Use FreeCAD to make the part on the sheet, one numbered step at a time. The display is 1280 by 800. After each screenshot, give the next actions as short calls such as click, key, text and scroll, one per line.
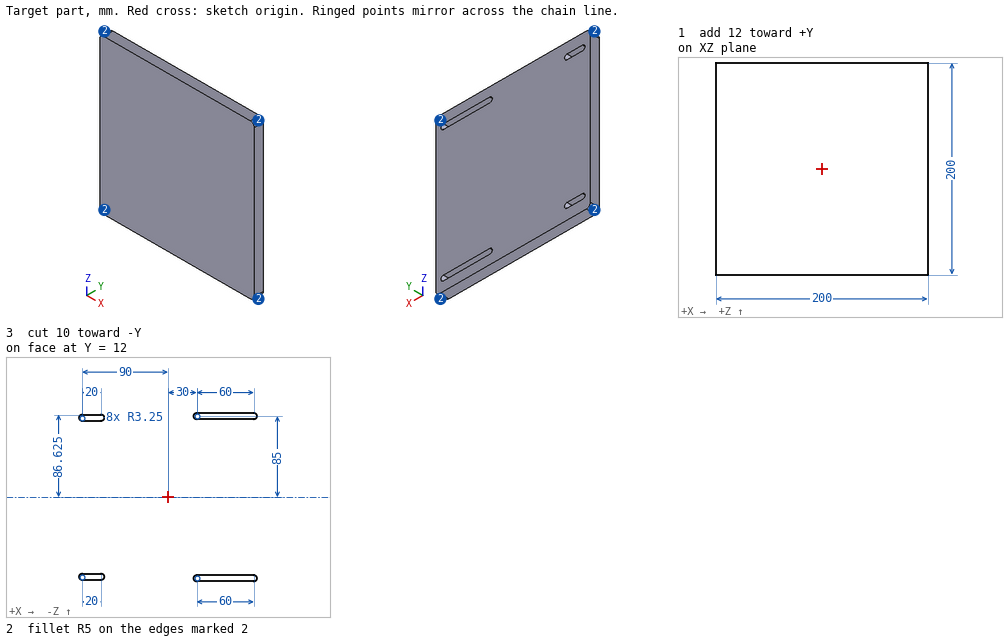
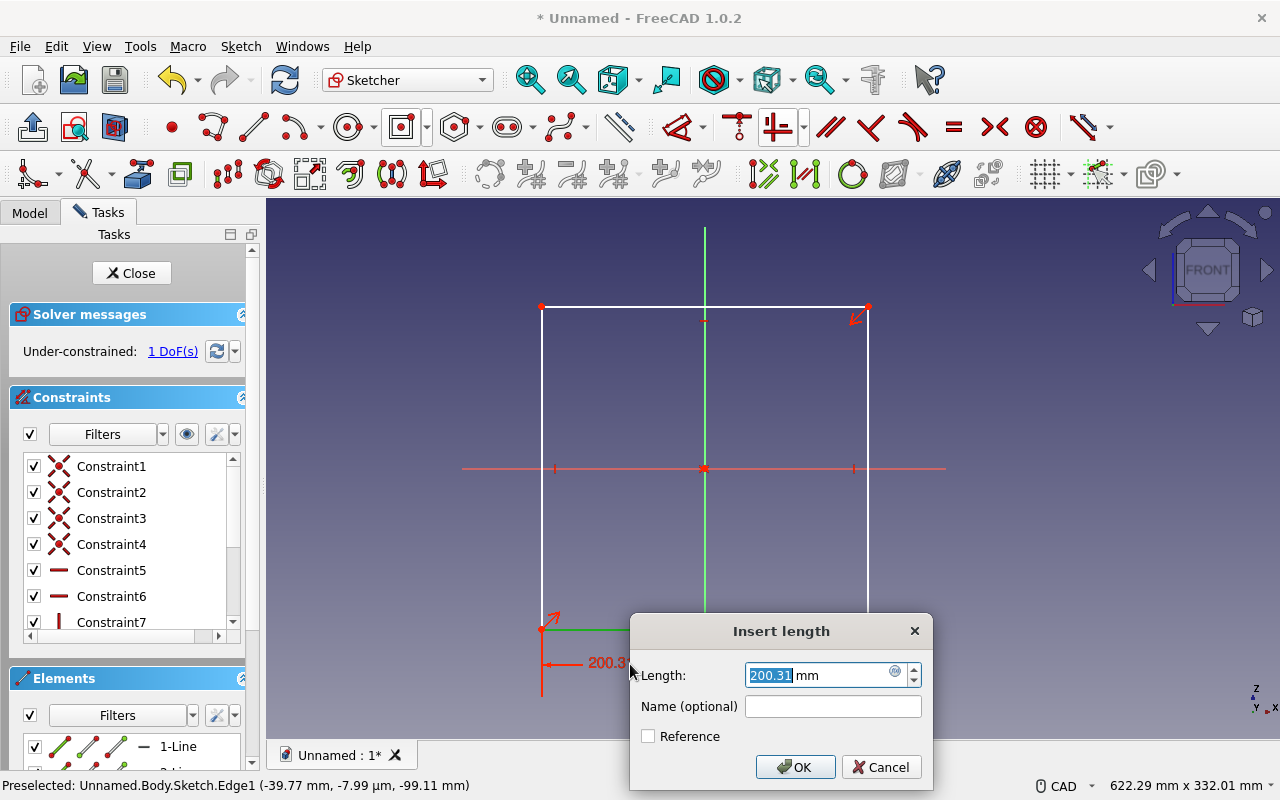
text(200)
key(Return)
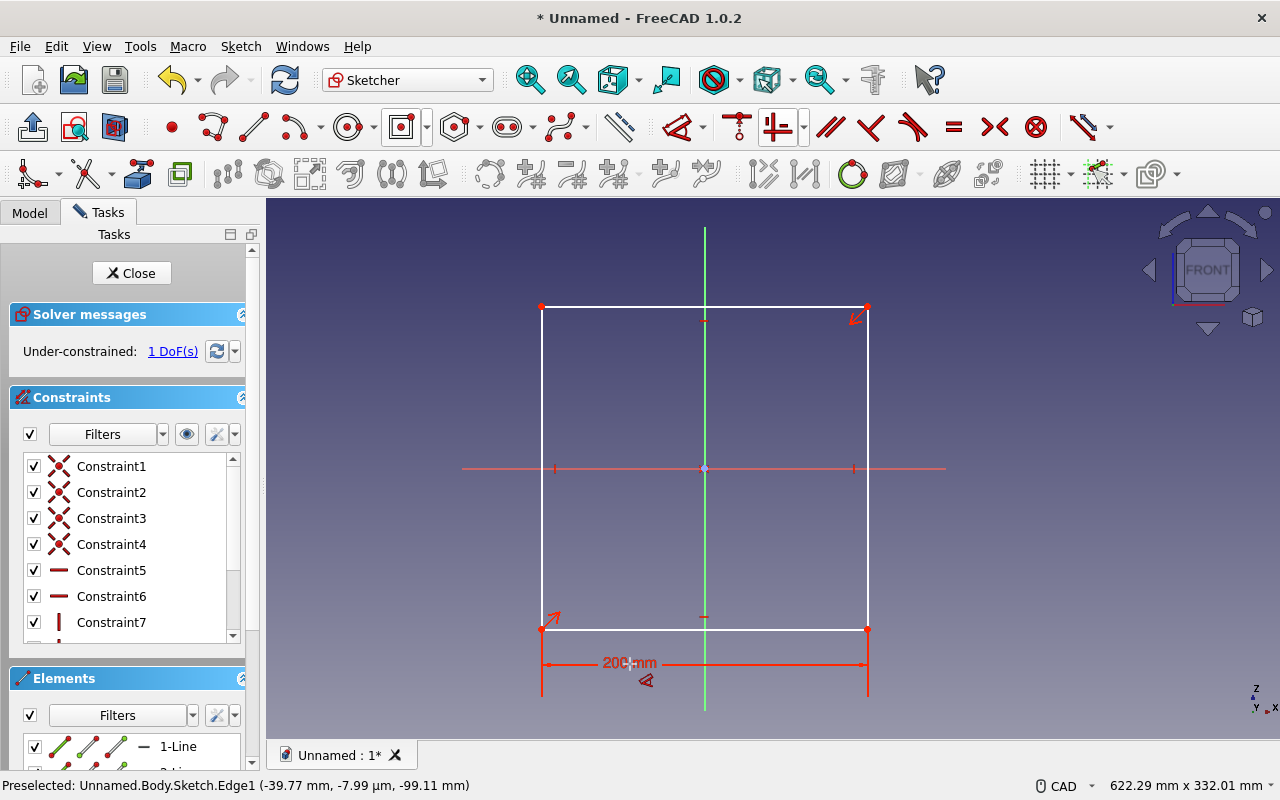
click(868, 533)
click(902, 394)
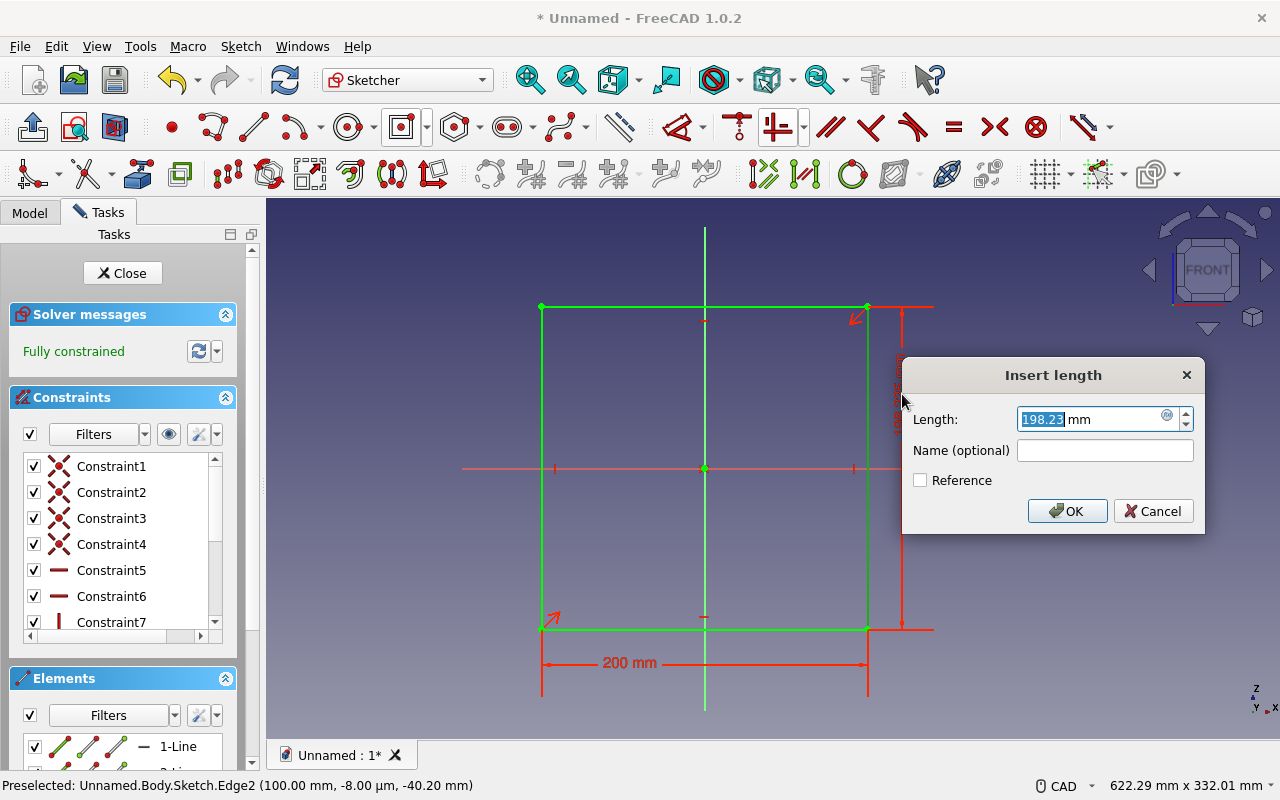
text(200)
key(Return)
key(Escape)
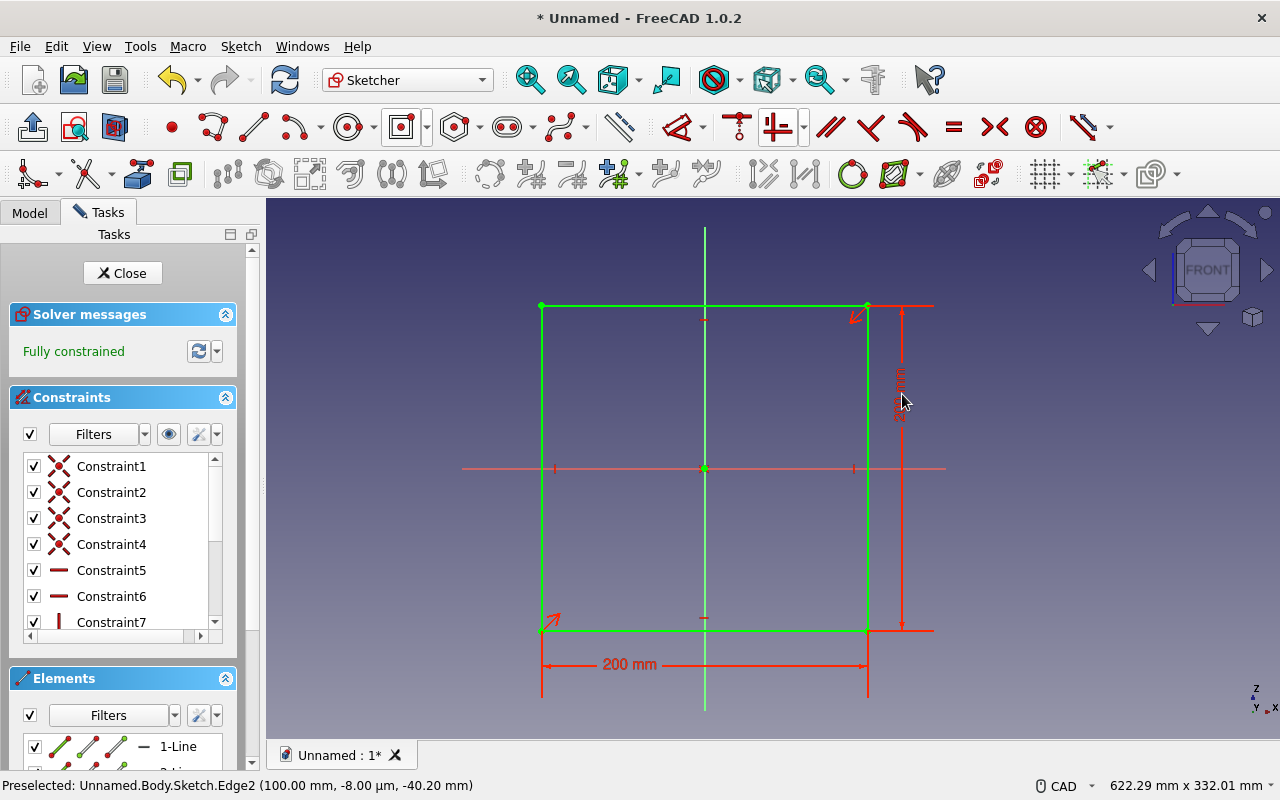
click(123, 273)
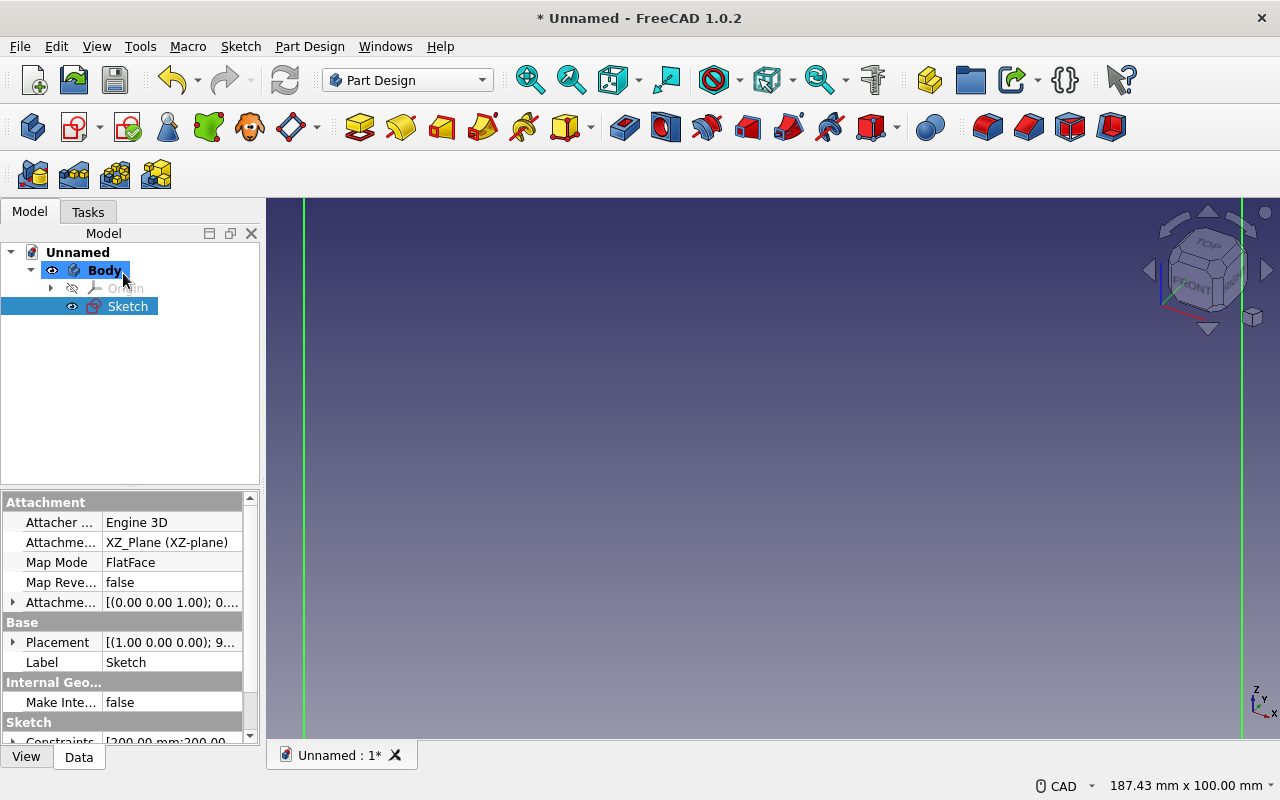
click(360, 128)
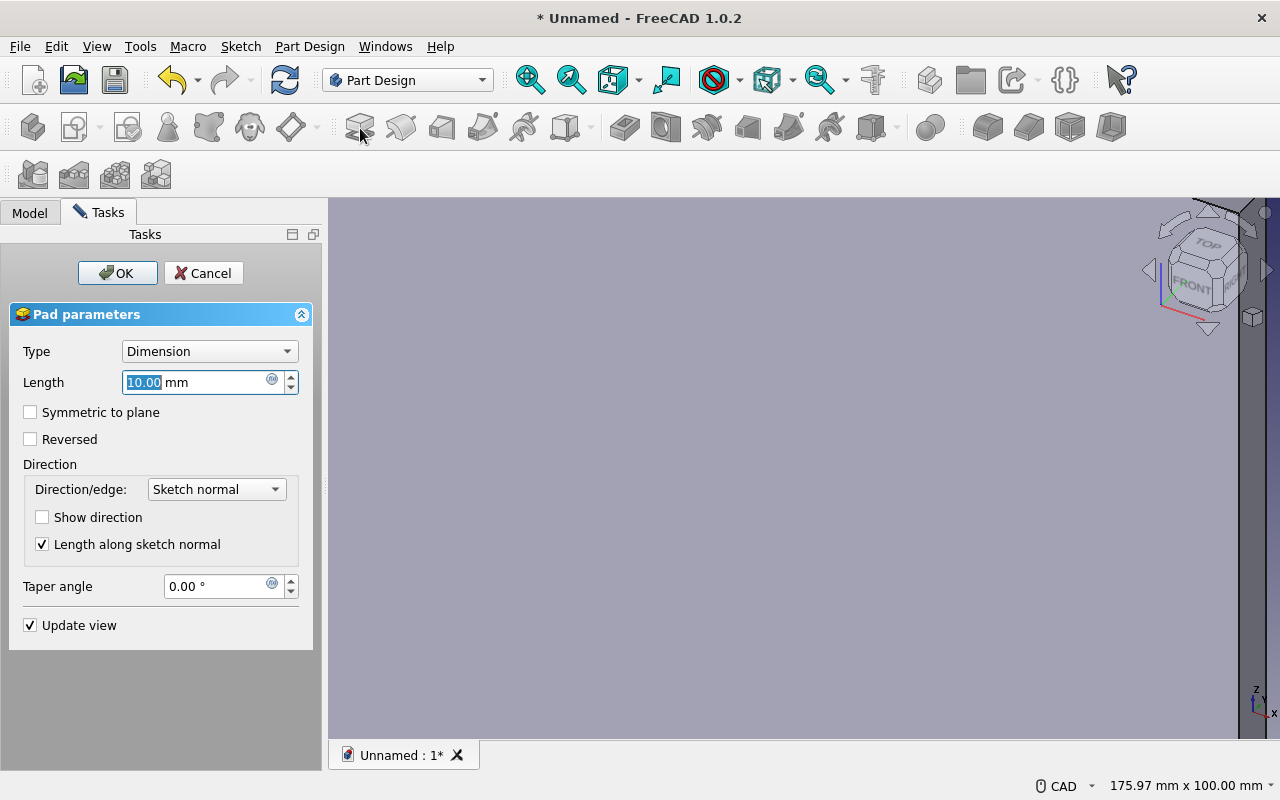
text(12)
key(Tab)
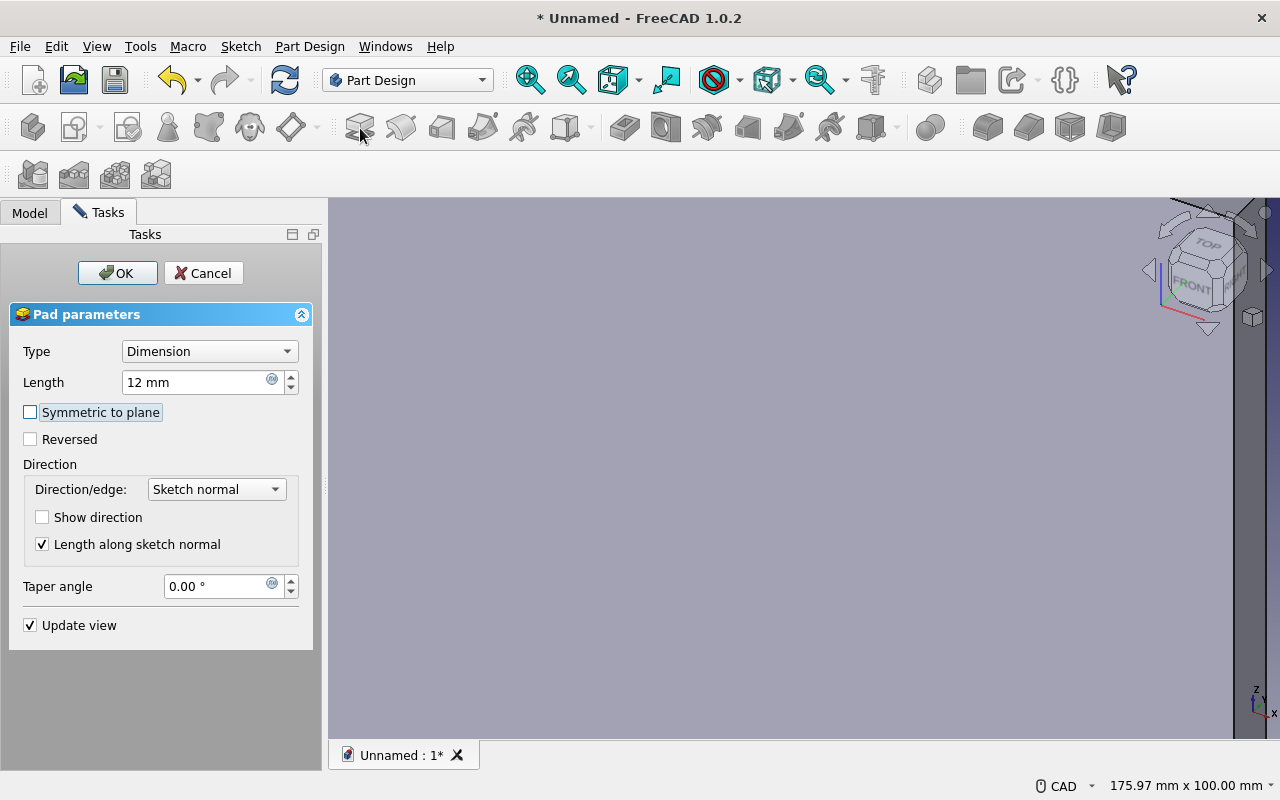
click(31, 439)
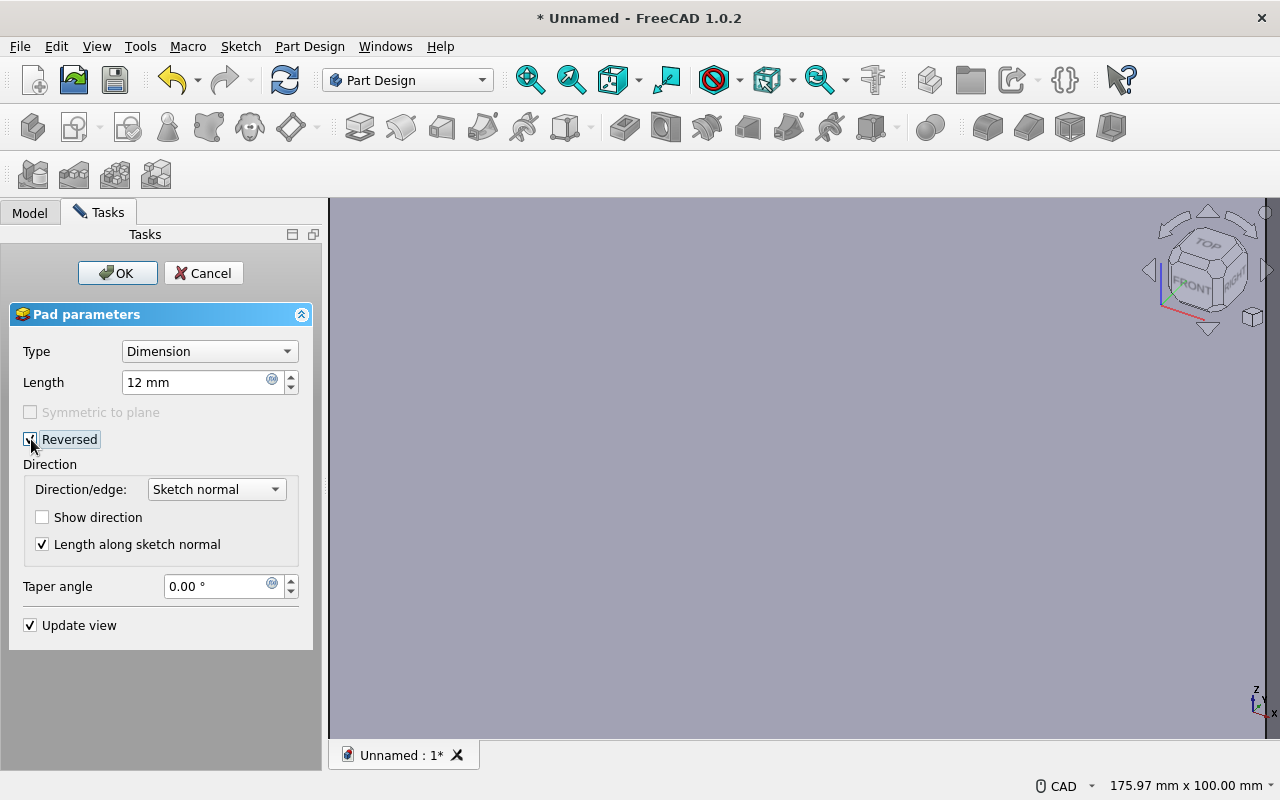
click(118, 273)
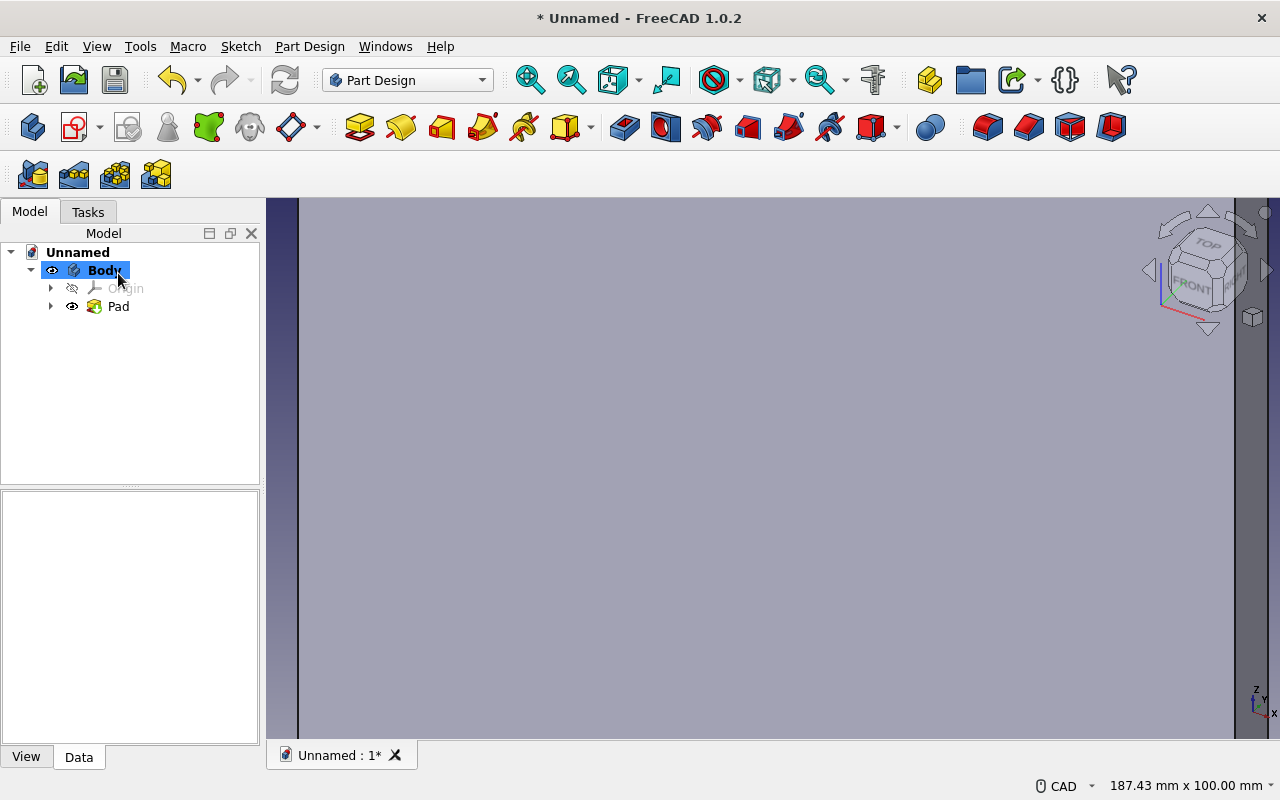
click(531, 80)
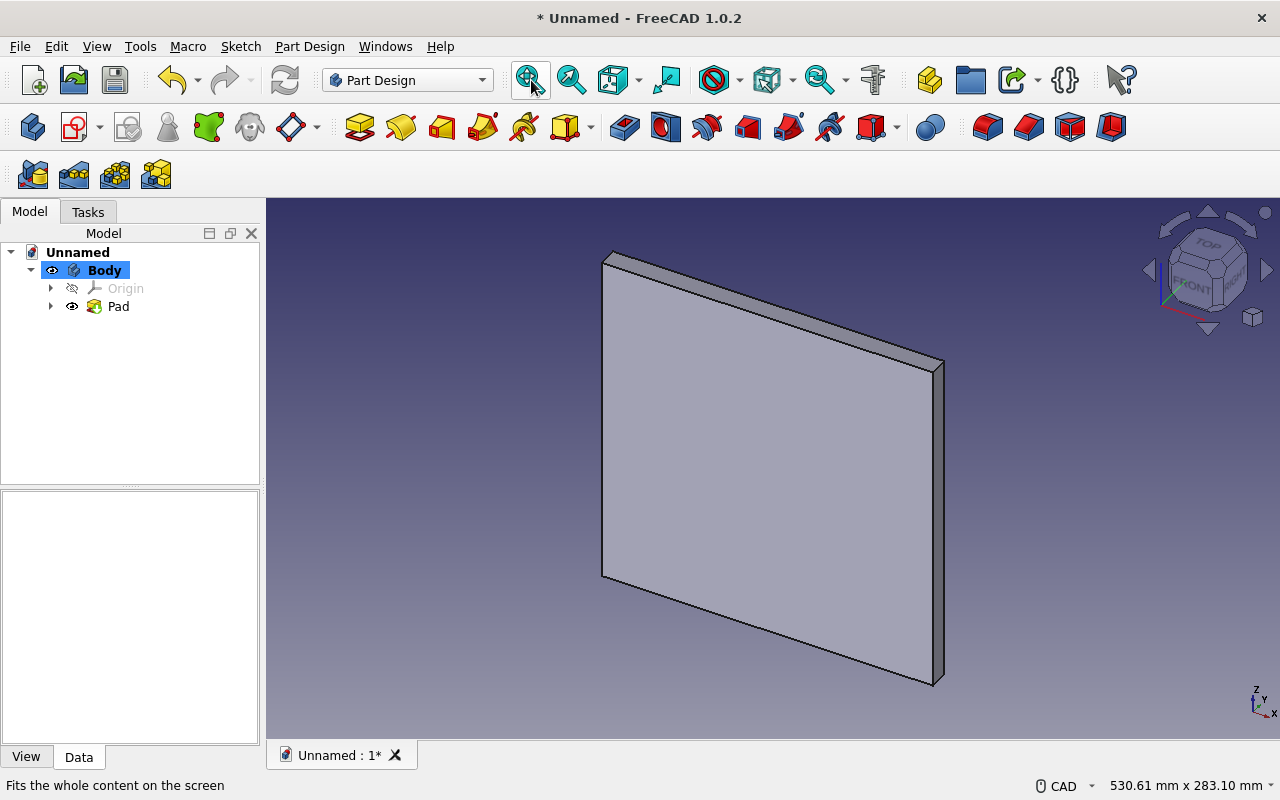
click(938, 366)